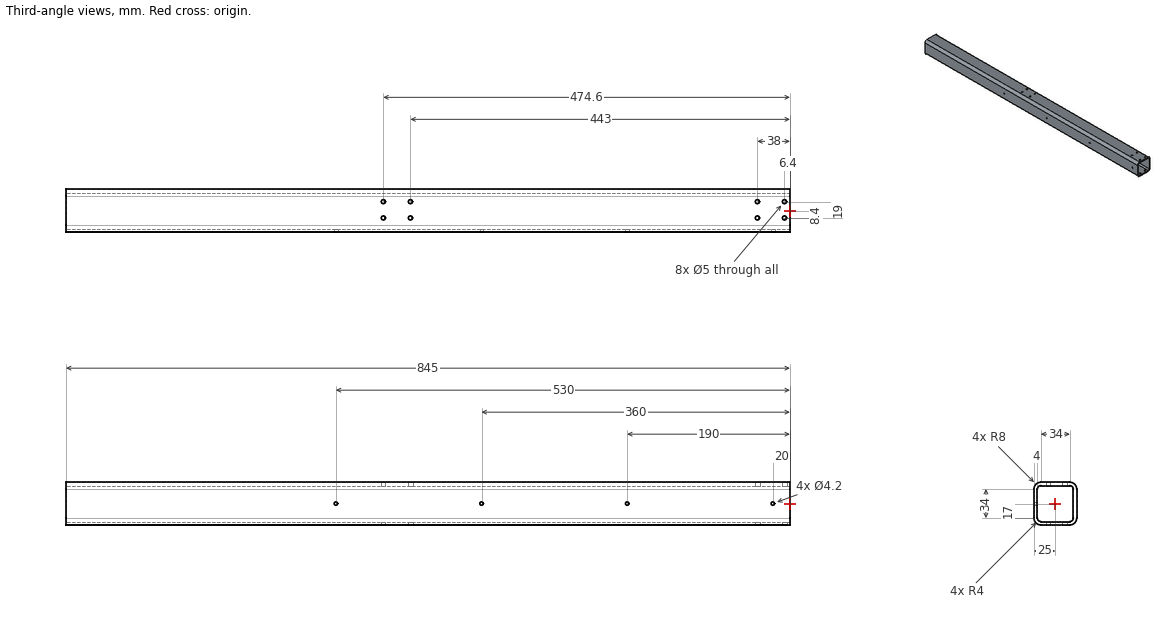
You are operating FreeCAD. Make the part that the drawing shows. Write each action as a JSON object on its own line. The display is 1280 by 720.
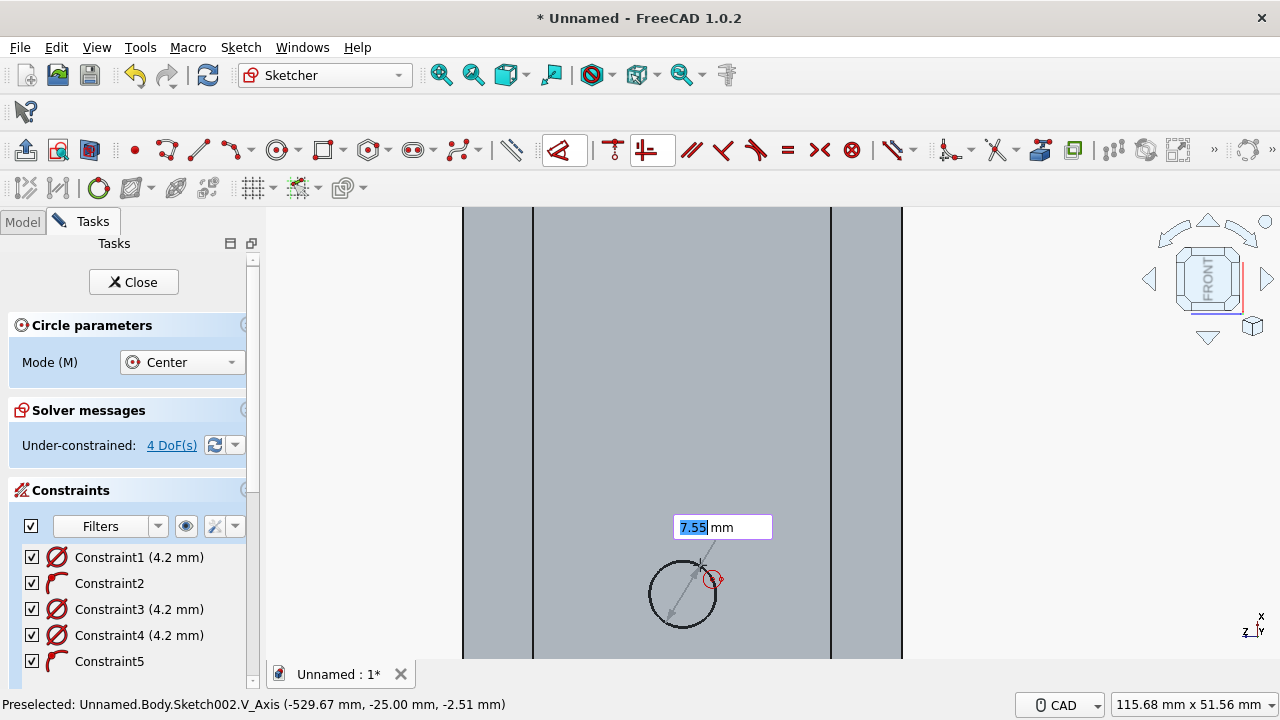
{"action": "type", "text": "4.2"}
{"action": "key", "text": "Return"}
{"action": "key", "text": "Escape"}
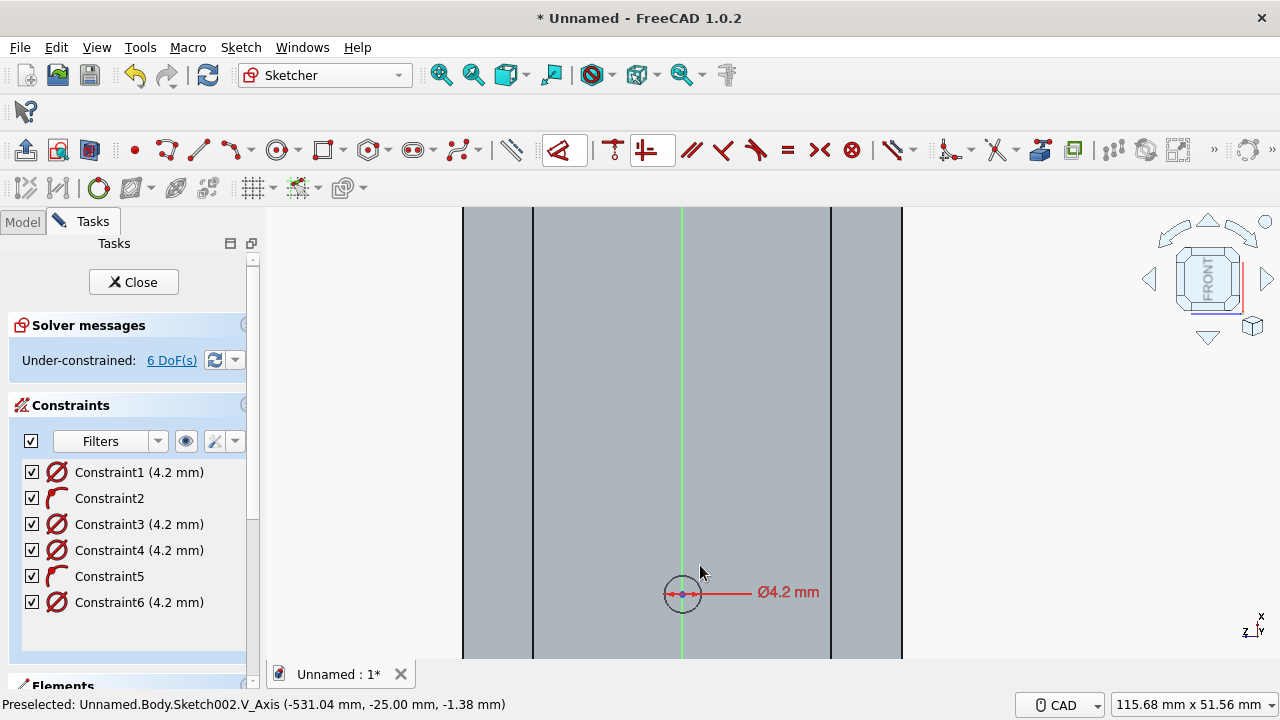
{"action": "scroll", "coordinate": [706, 574], "scroll_direction": "down", "scroll_amount": 14}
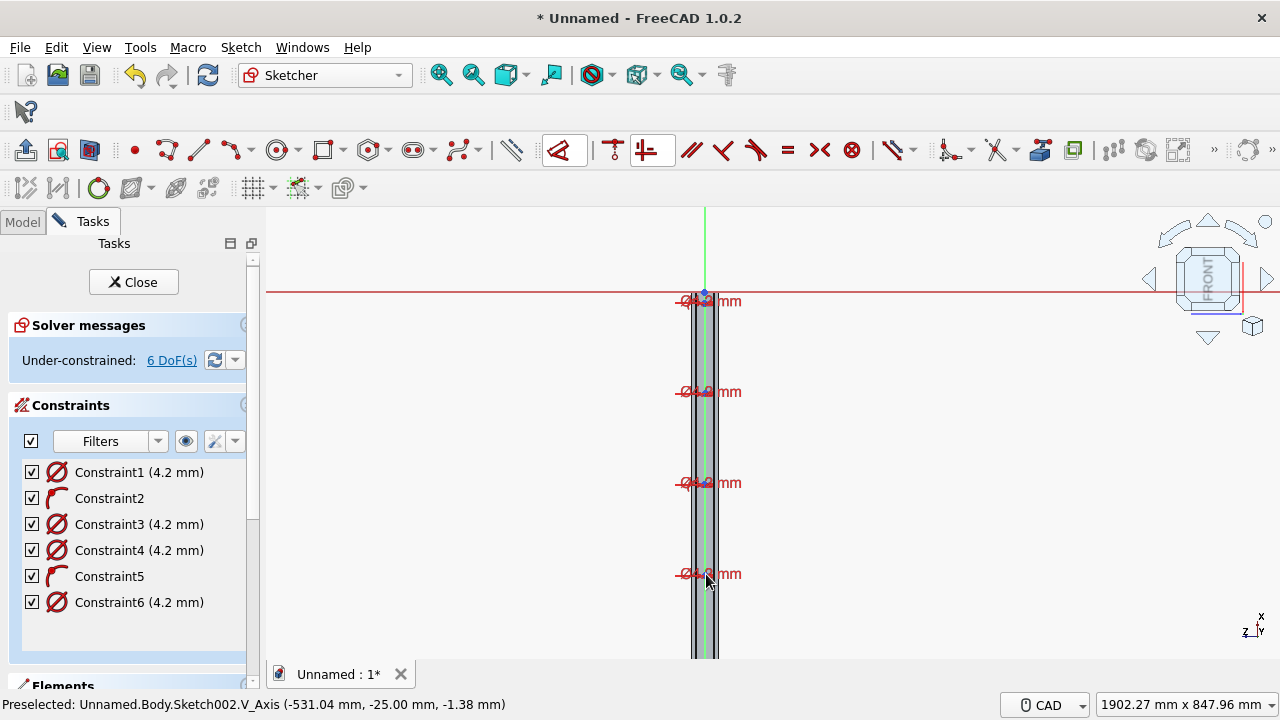
{"action": "left_click", "coordinate": [705, 394]}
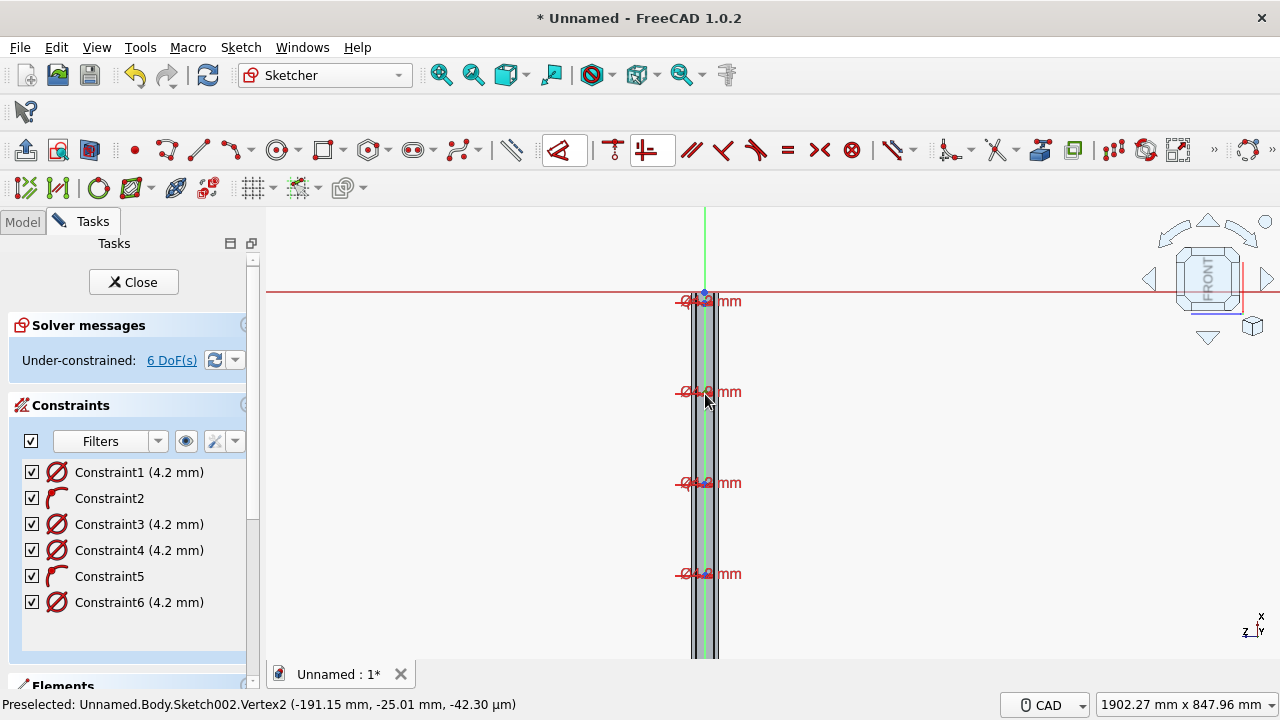
{"action": "left_click", "coordinate": [705, 518]}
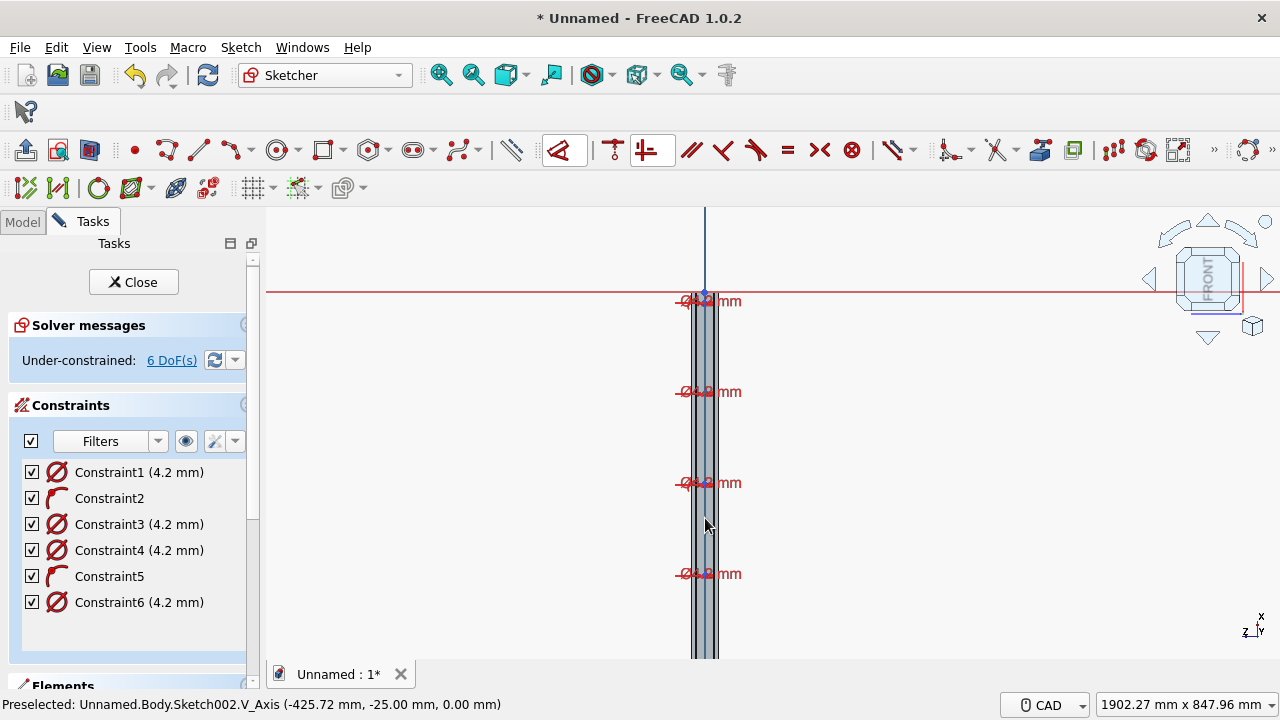
{"action": "left_click", "coordinate": [614, 150]}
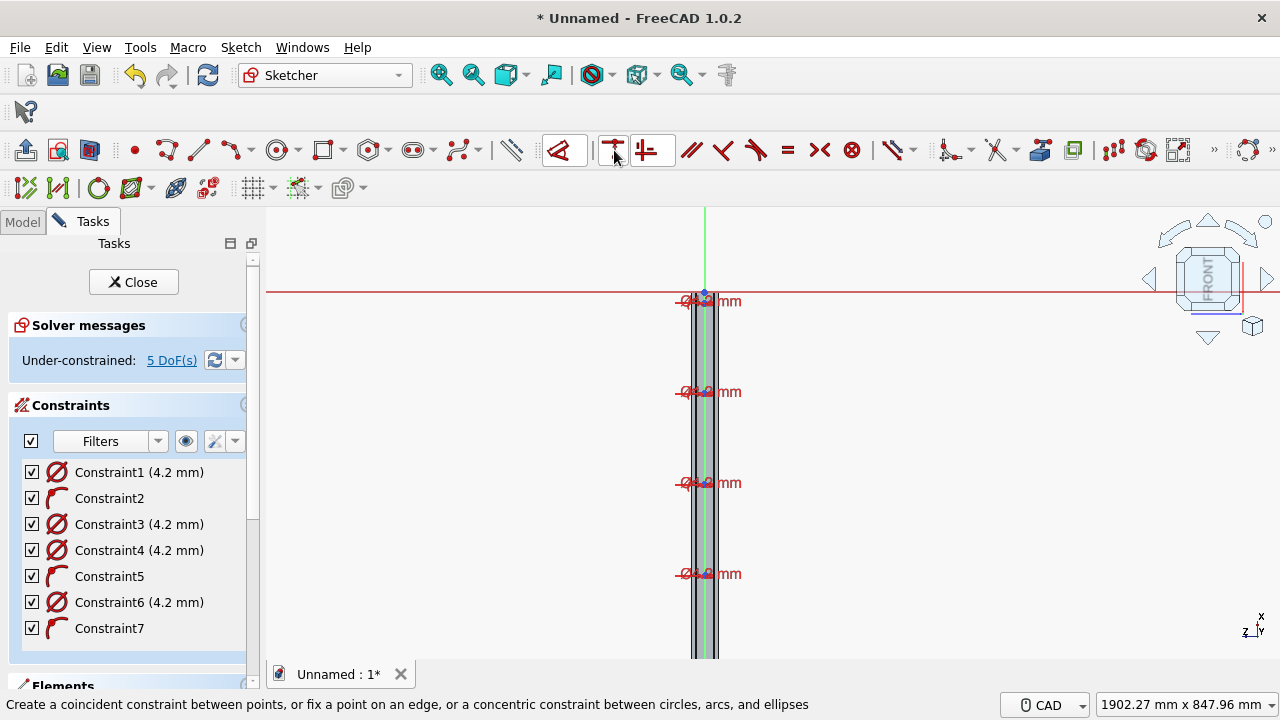
{"action": "left_click", "coordinate": [705, 576]}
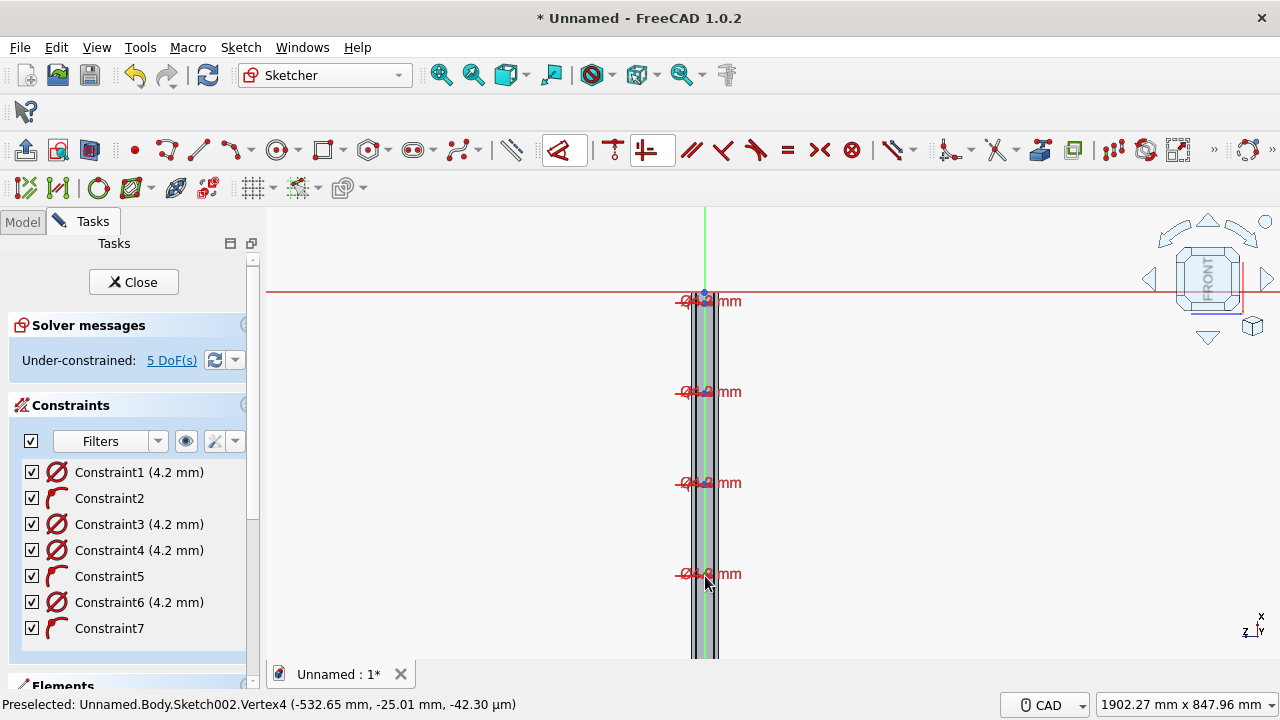
{"action": "left_click", "coordinate": [705, 518]}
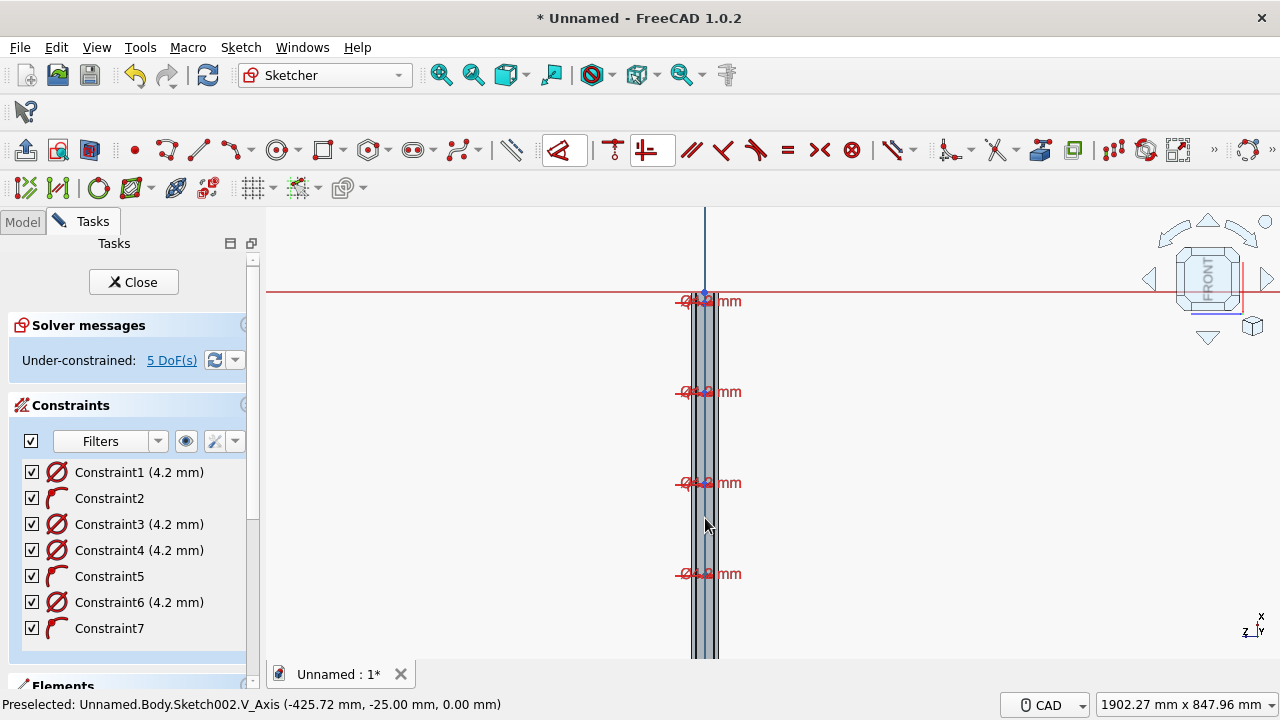
{"action": "left_click", "coordinate": [614, 150]}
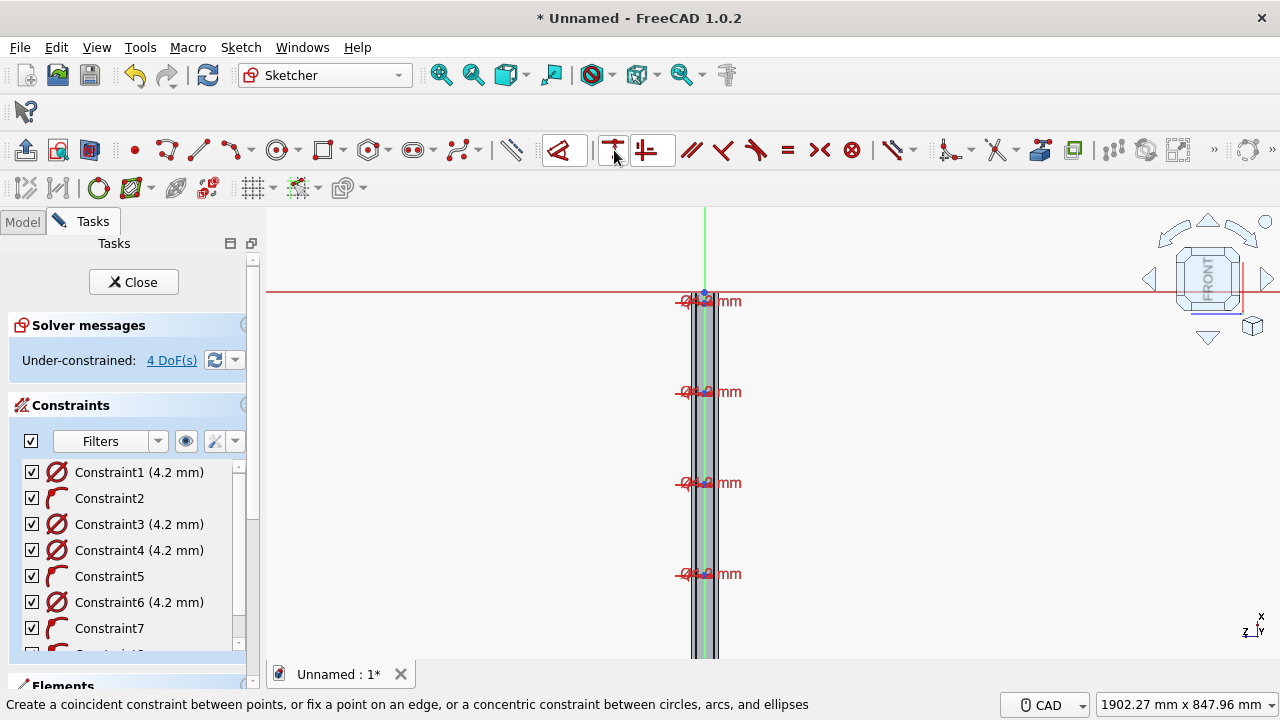
{"action": "scroll", "coordinate": [705, 303], "scroll_direction": "up", "scroll_amount": 7}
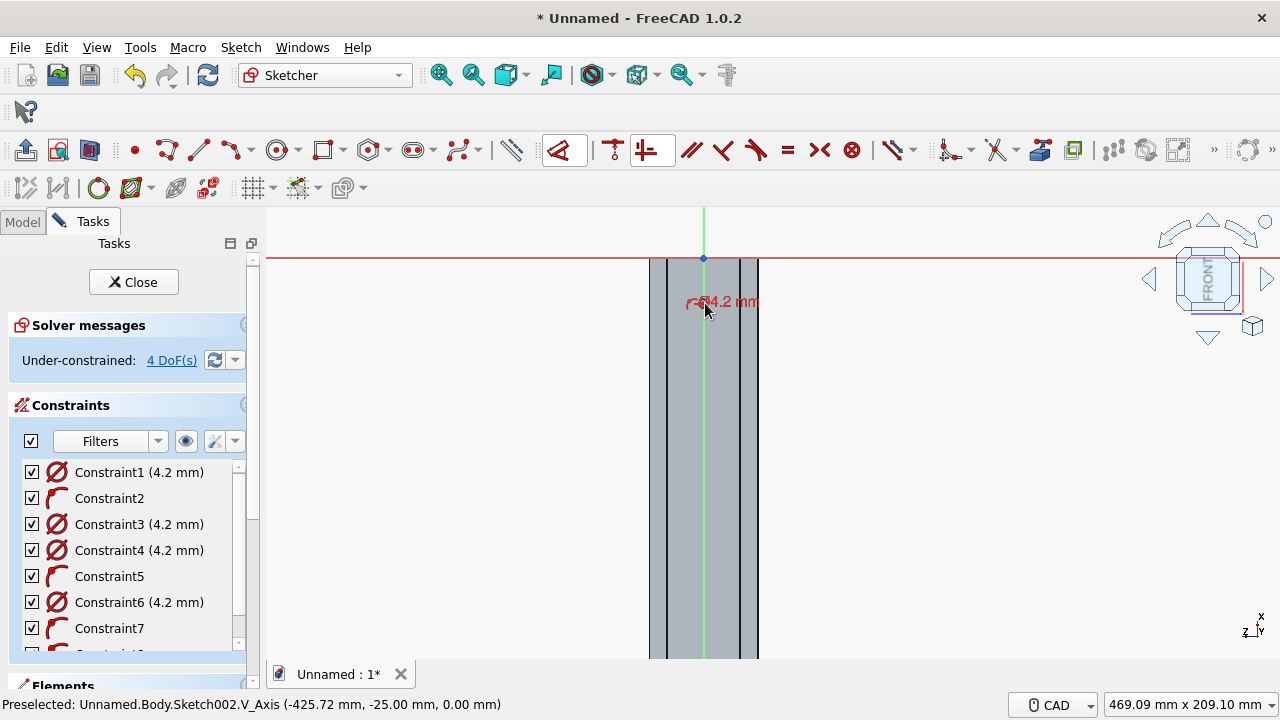
{"action": "left_click", "coordinate": [704, 304]}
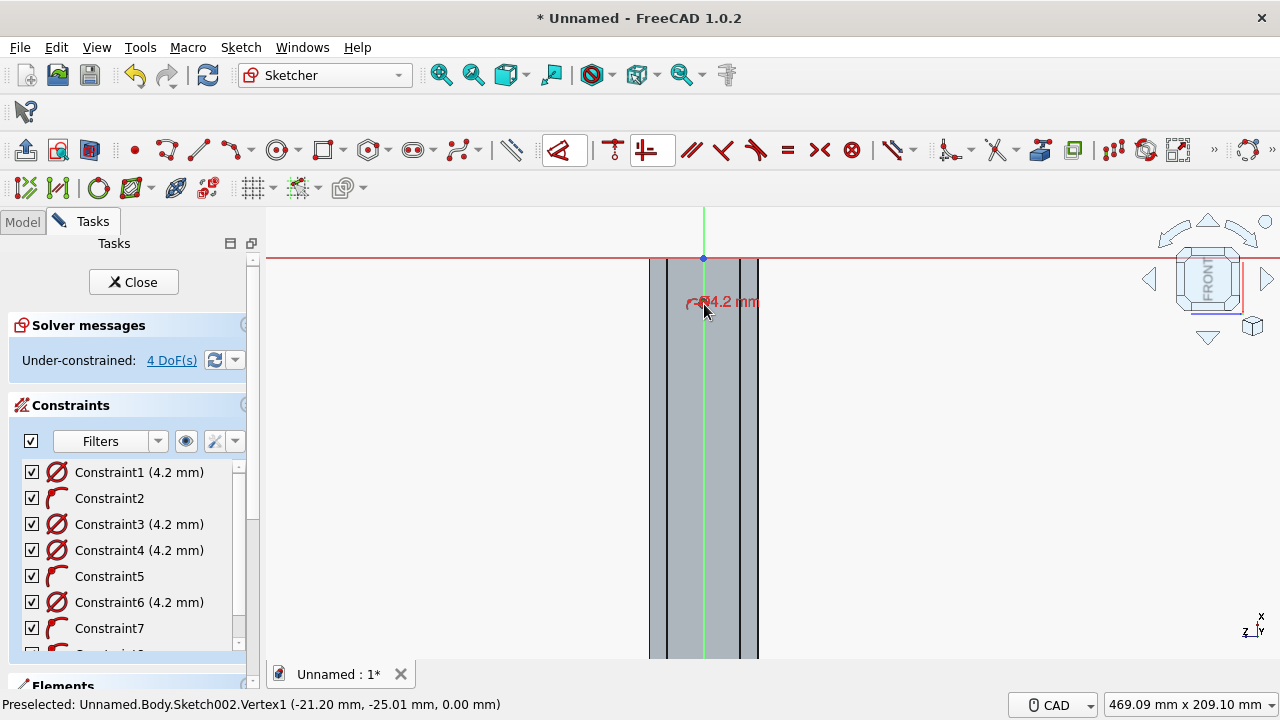
{"action": "left_click", "coordinate": [582, 150]}